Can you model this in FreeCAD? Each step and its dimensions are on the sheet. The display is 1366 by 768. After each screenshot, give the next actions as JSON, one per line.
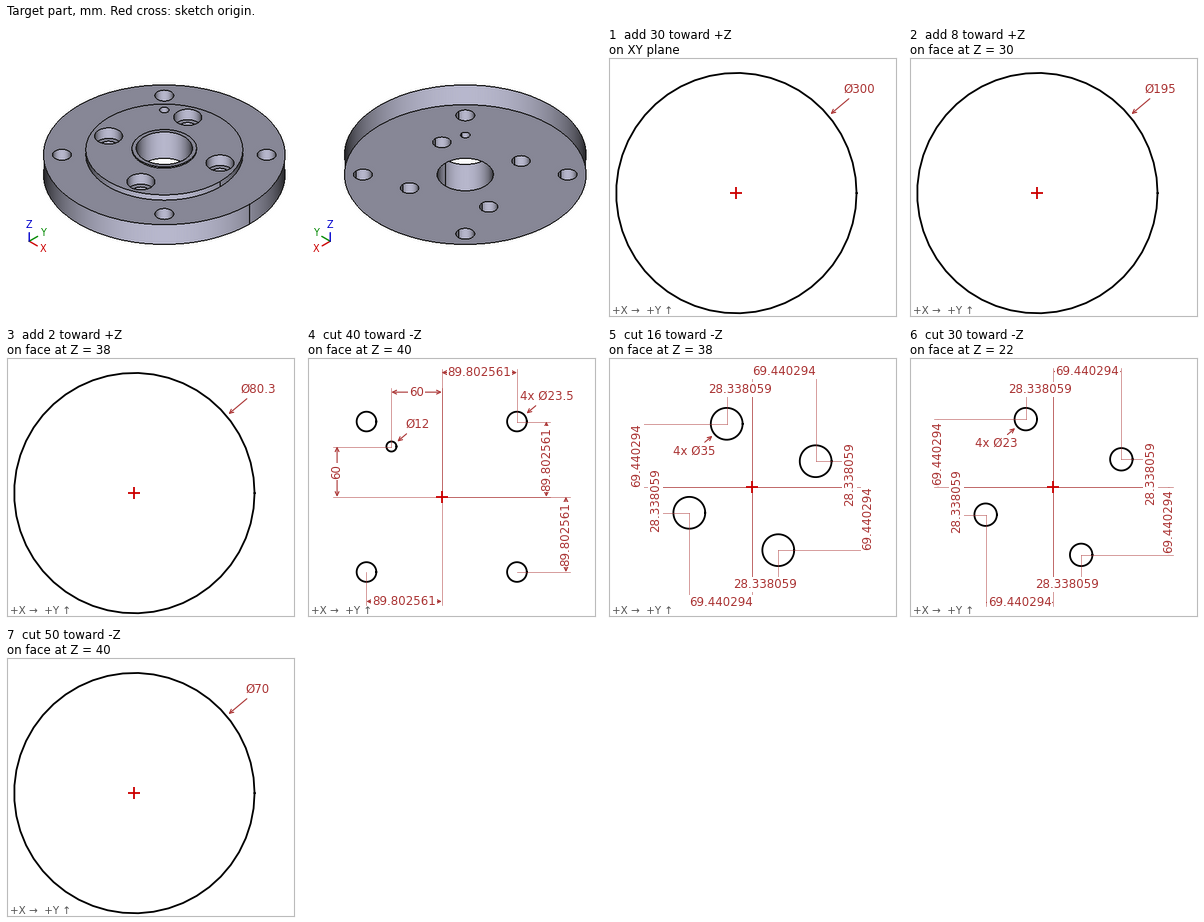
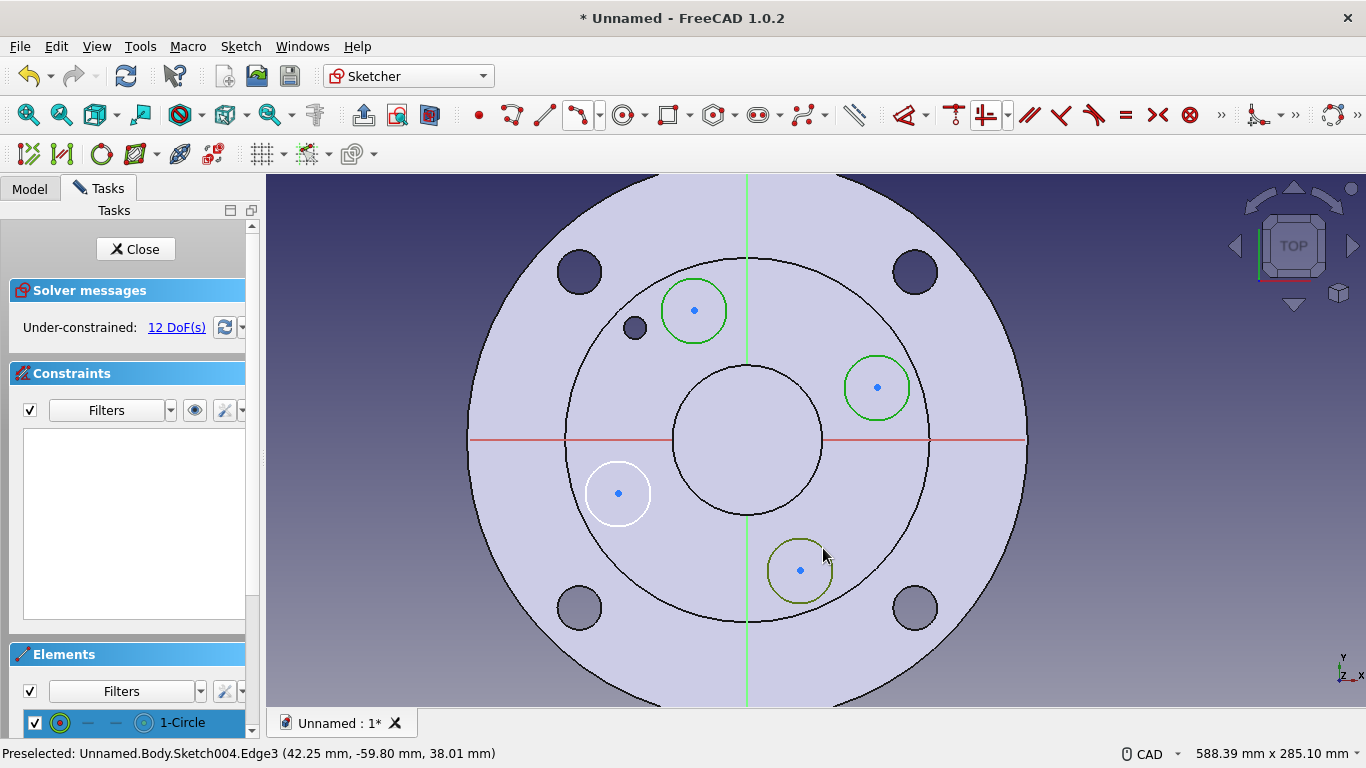
{"action": "left_click", "coordinate": [641, 471]}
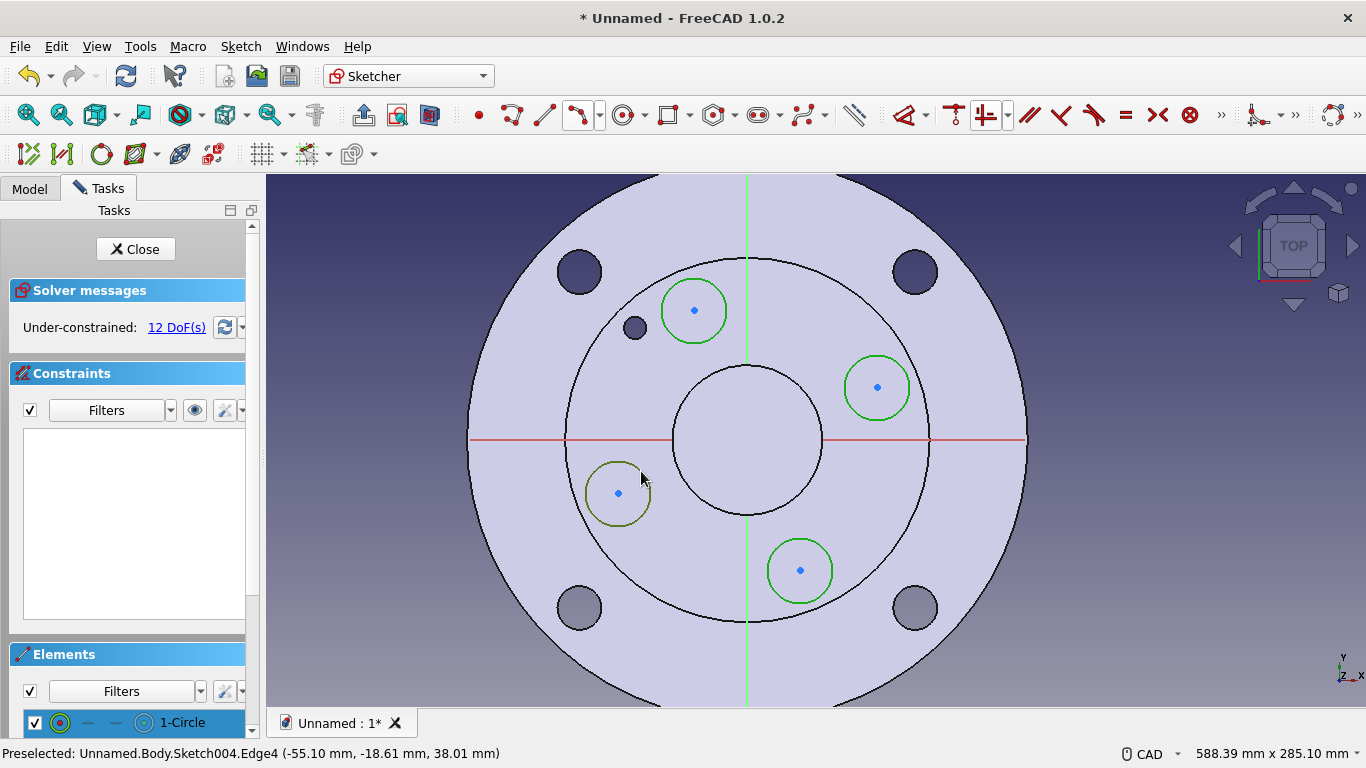
{"action": "key", "text": "e"}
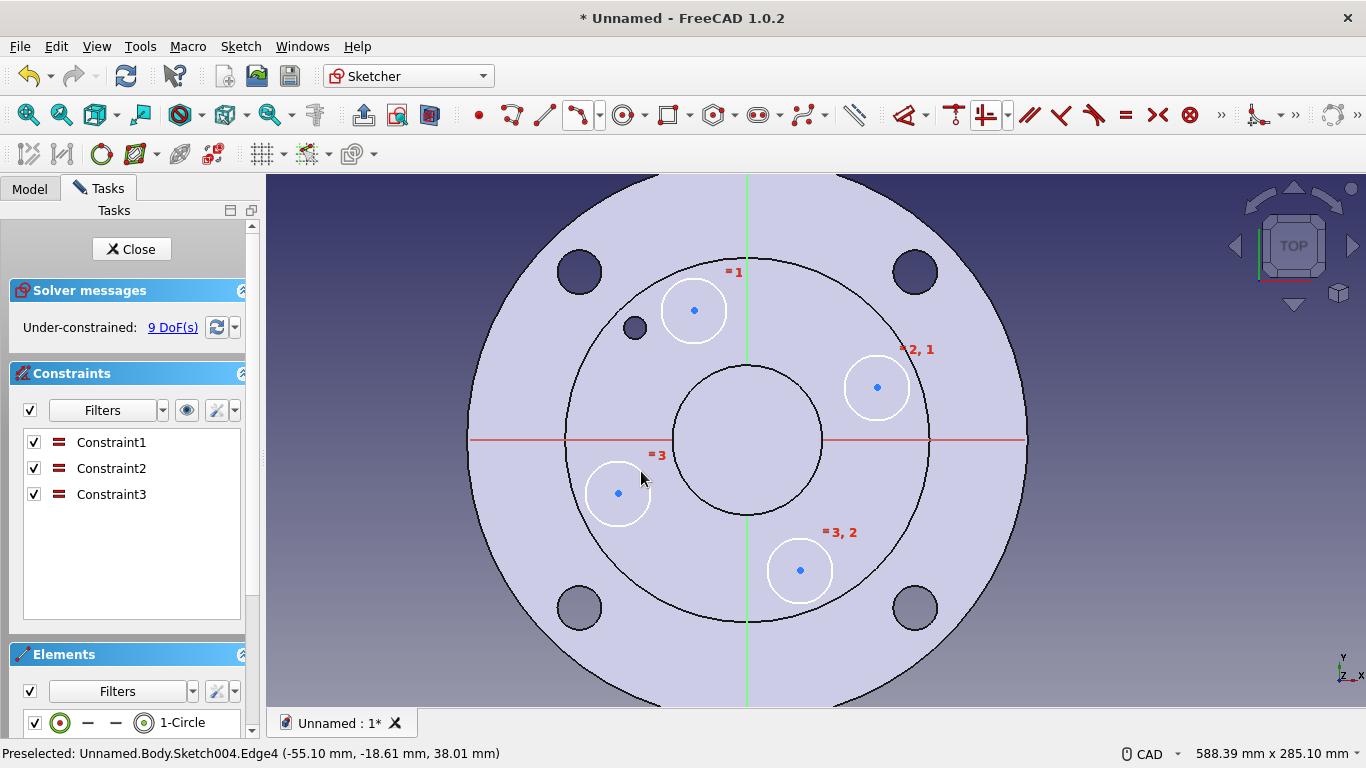
{"action": "key", "text": "d"}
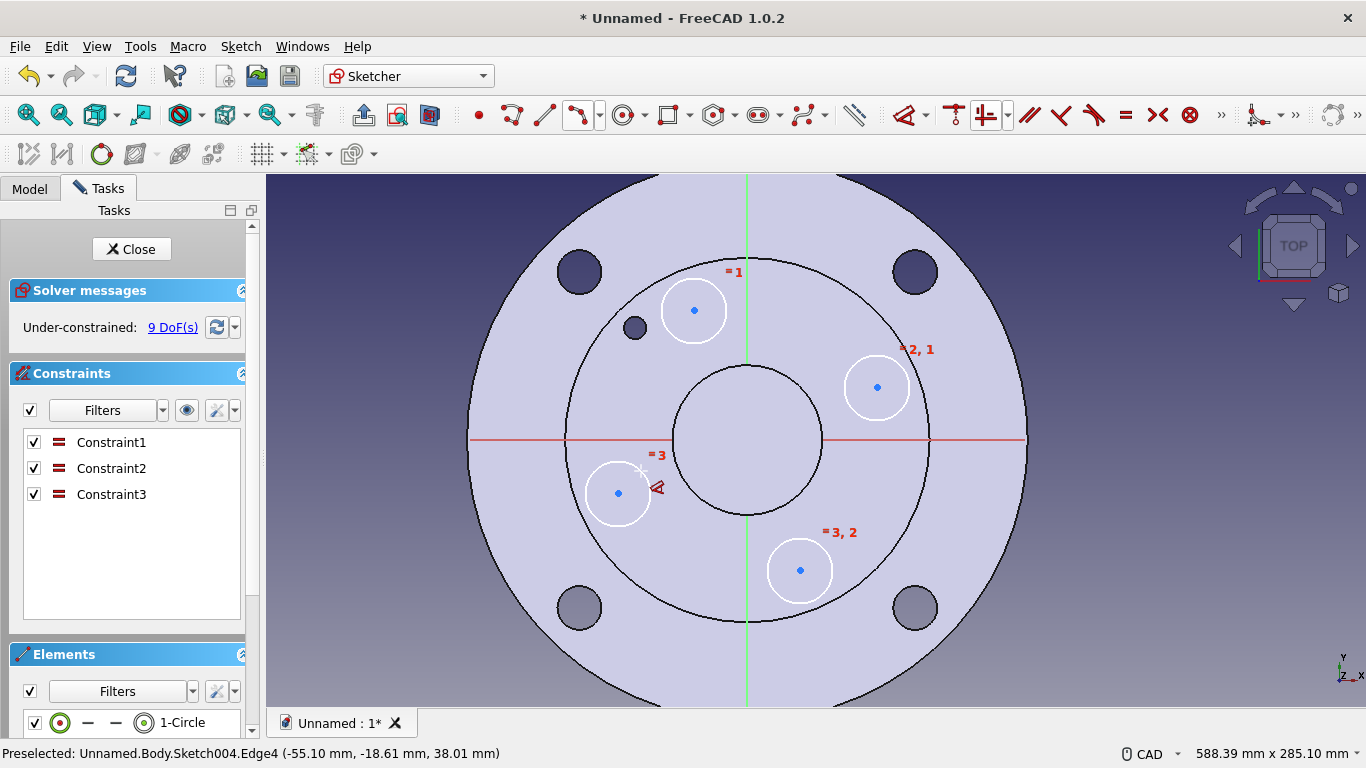
{"action": "left_click", "coordinate": [717, 288]}
{"action": "left_click", "coordinate": [712, 249]}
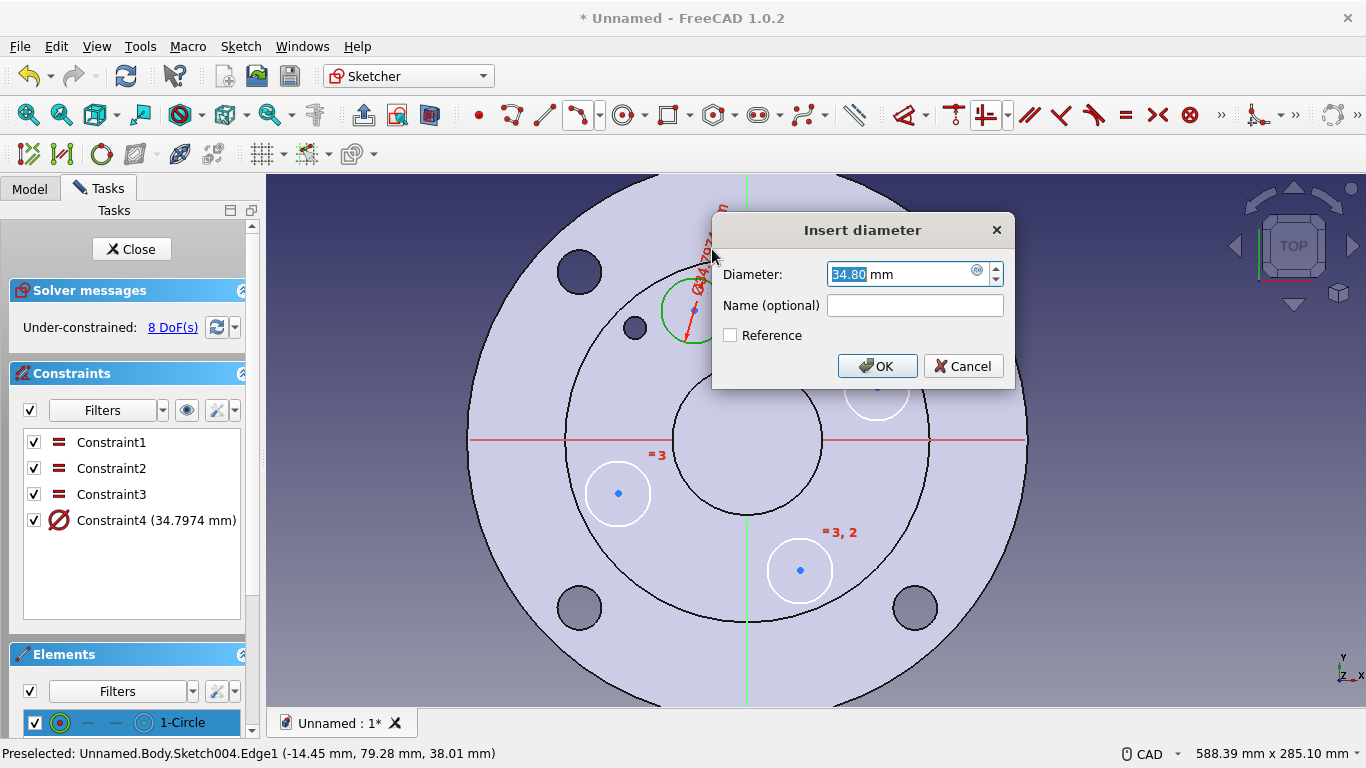
{"action": "type", "text": "35"}
{"action": "key", "text": "Return"}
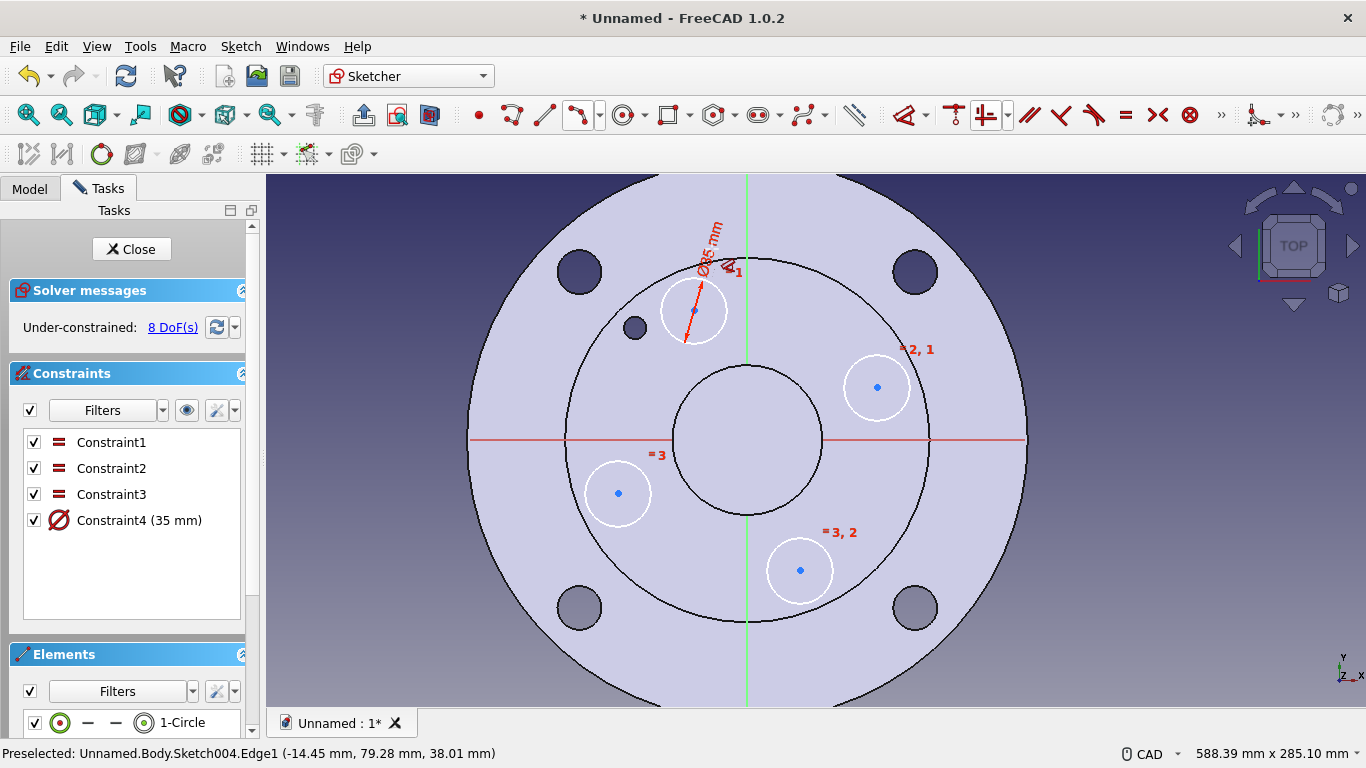
{"action": "left_click", "coordinate": [694, 311]}
{"action": "left_click", "coordinate": [733, 277]}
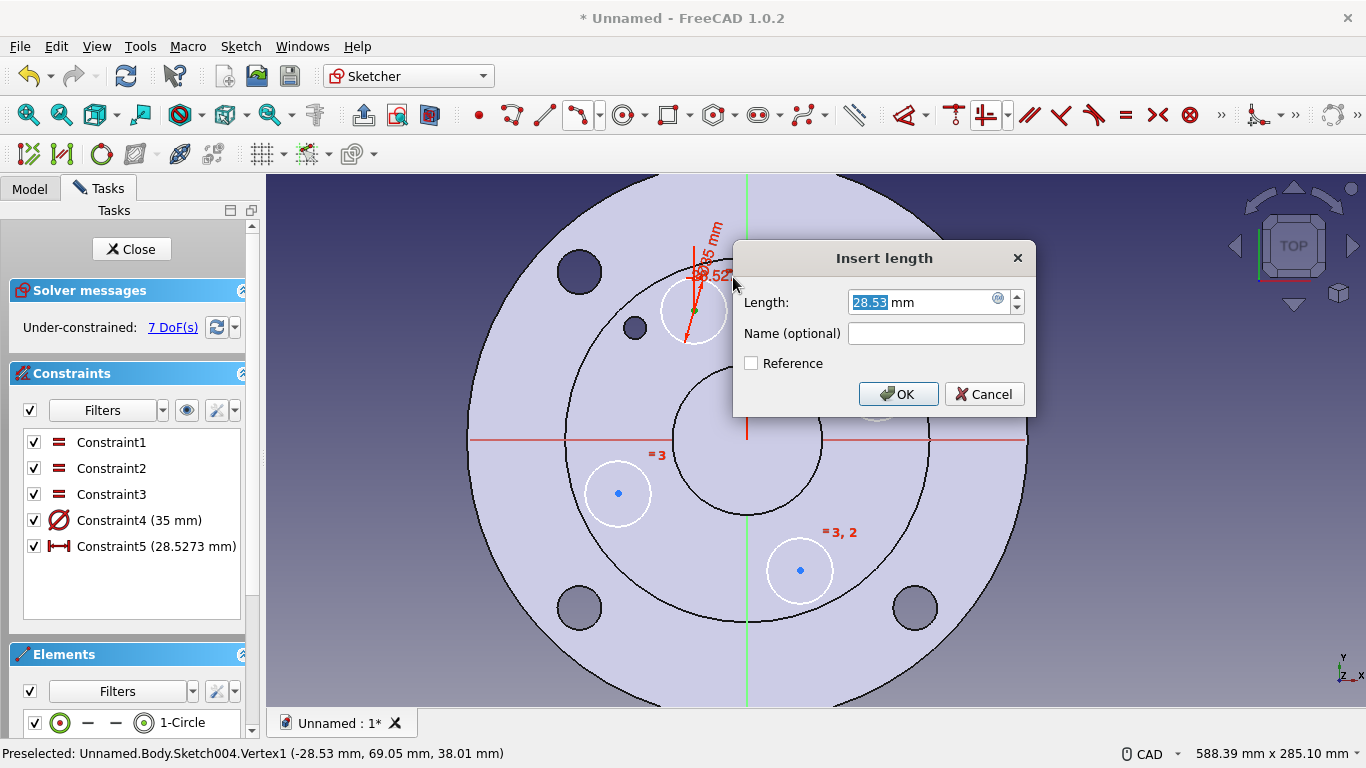
{"action": "type", "text": "28.338059"}
{"action": "key", "text": "Return"}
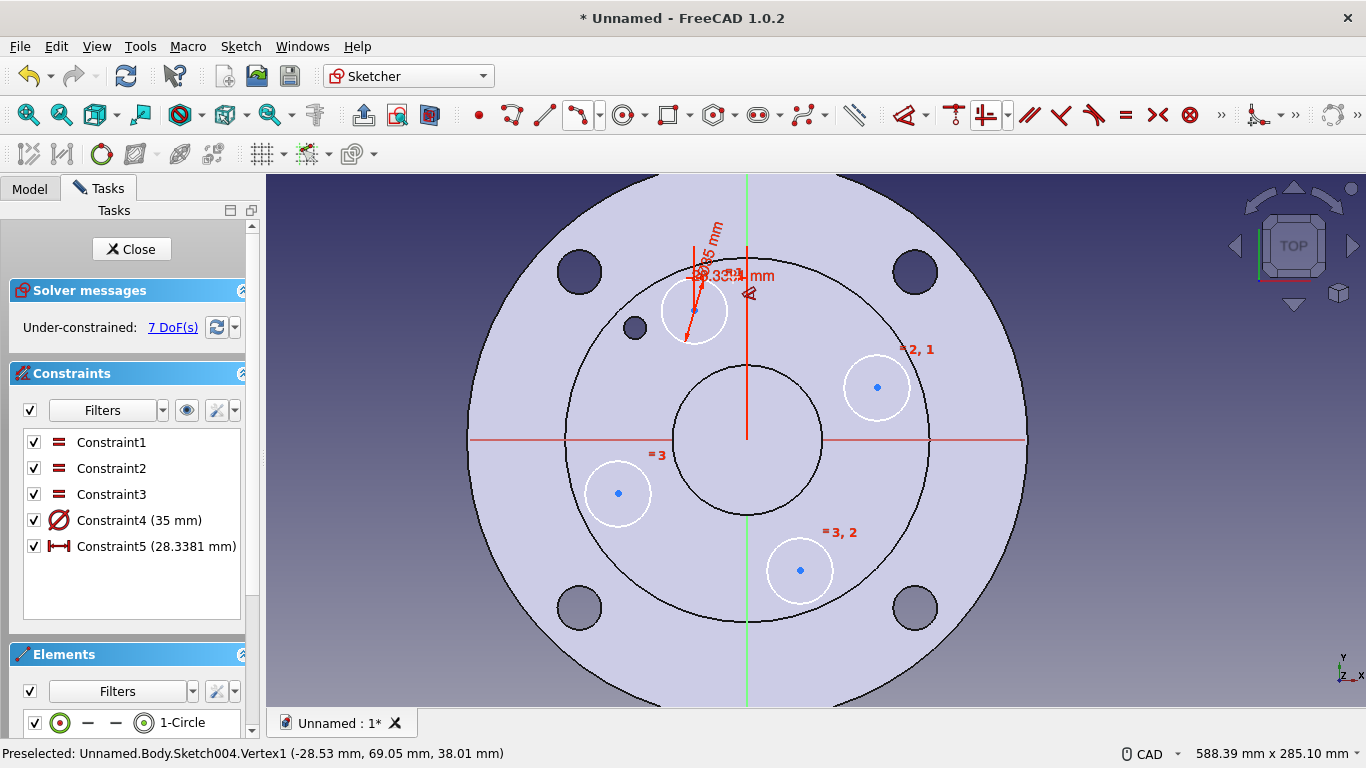
{"action": "left_click", "coordinate": [694, 311]}
{"action": "left_click", "coordinate": [660, 376]}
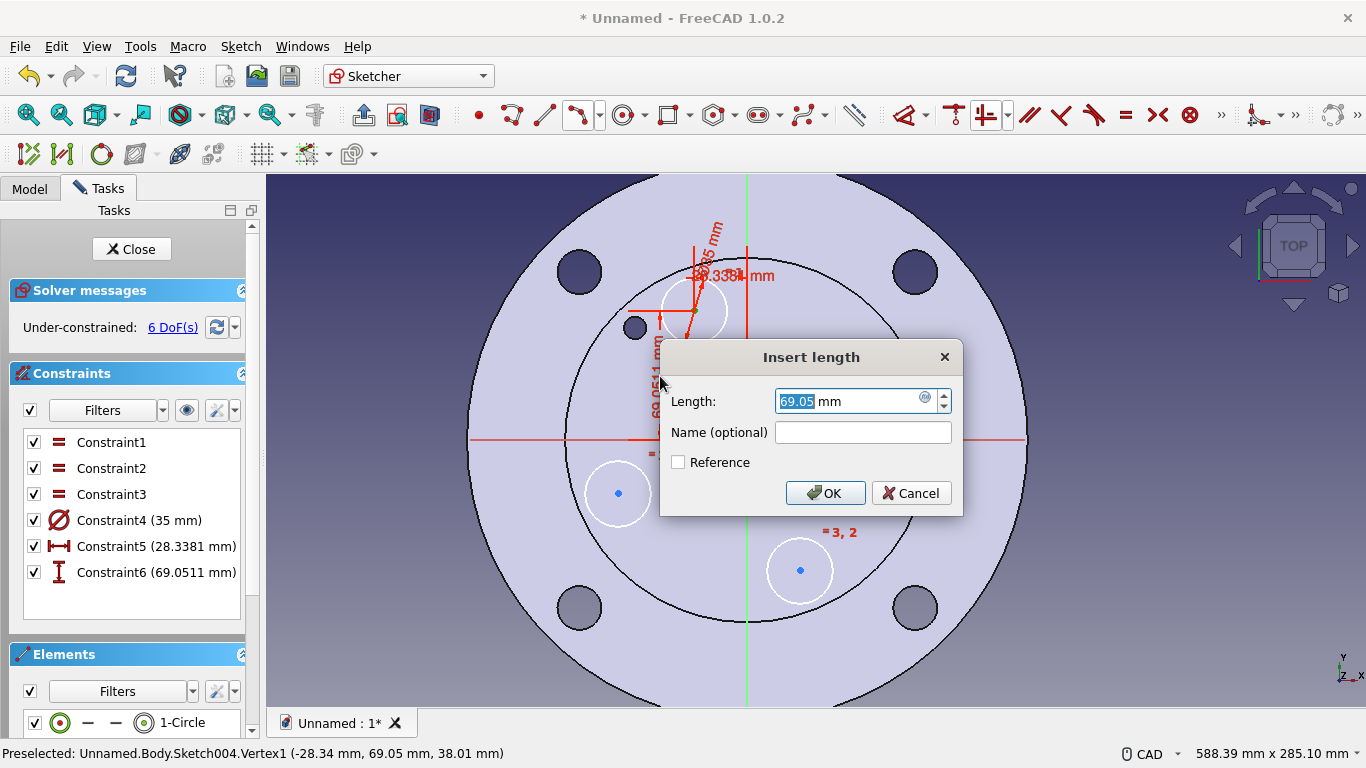
{"action": "type", "text": "69.440294"}
{"action": "key", "text": "Return"}